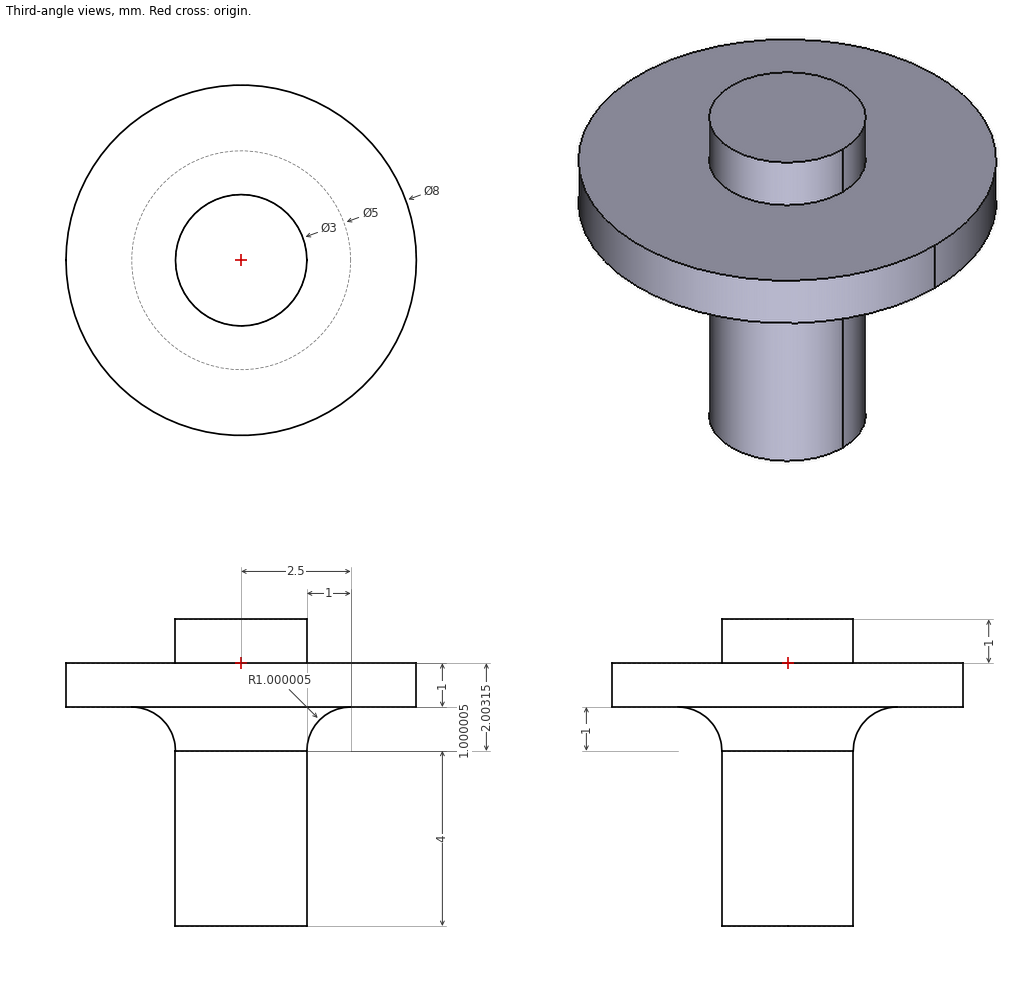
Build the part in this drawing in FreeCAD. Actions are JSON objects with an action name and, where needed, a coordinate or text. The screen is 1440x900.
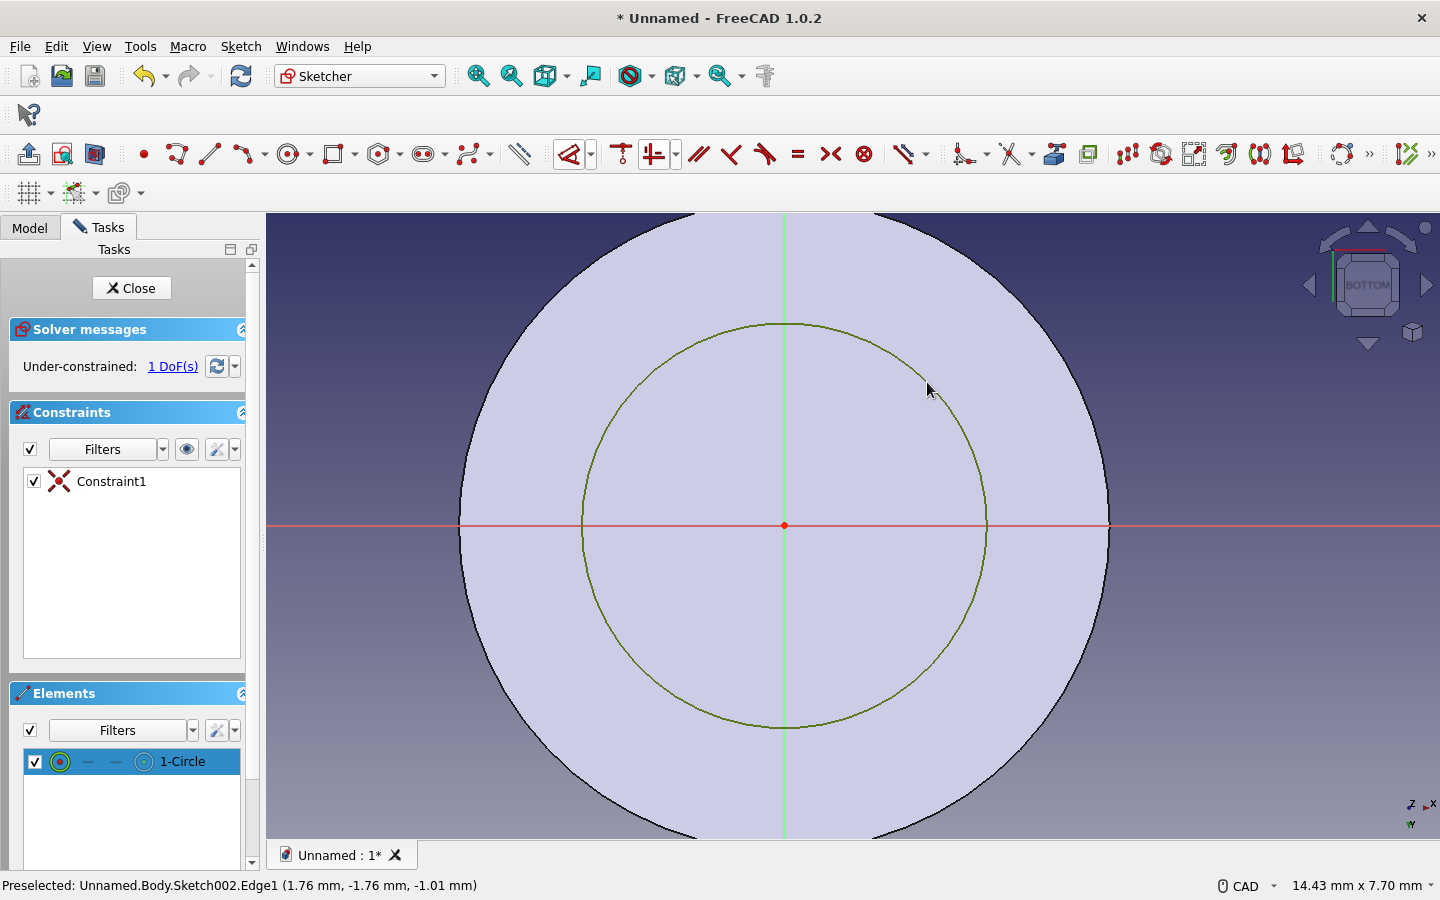
{"action": "key", "text": "k o"}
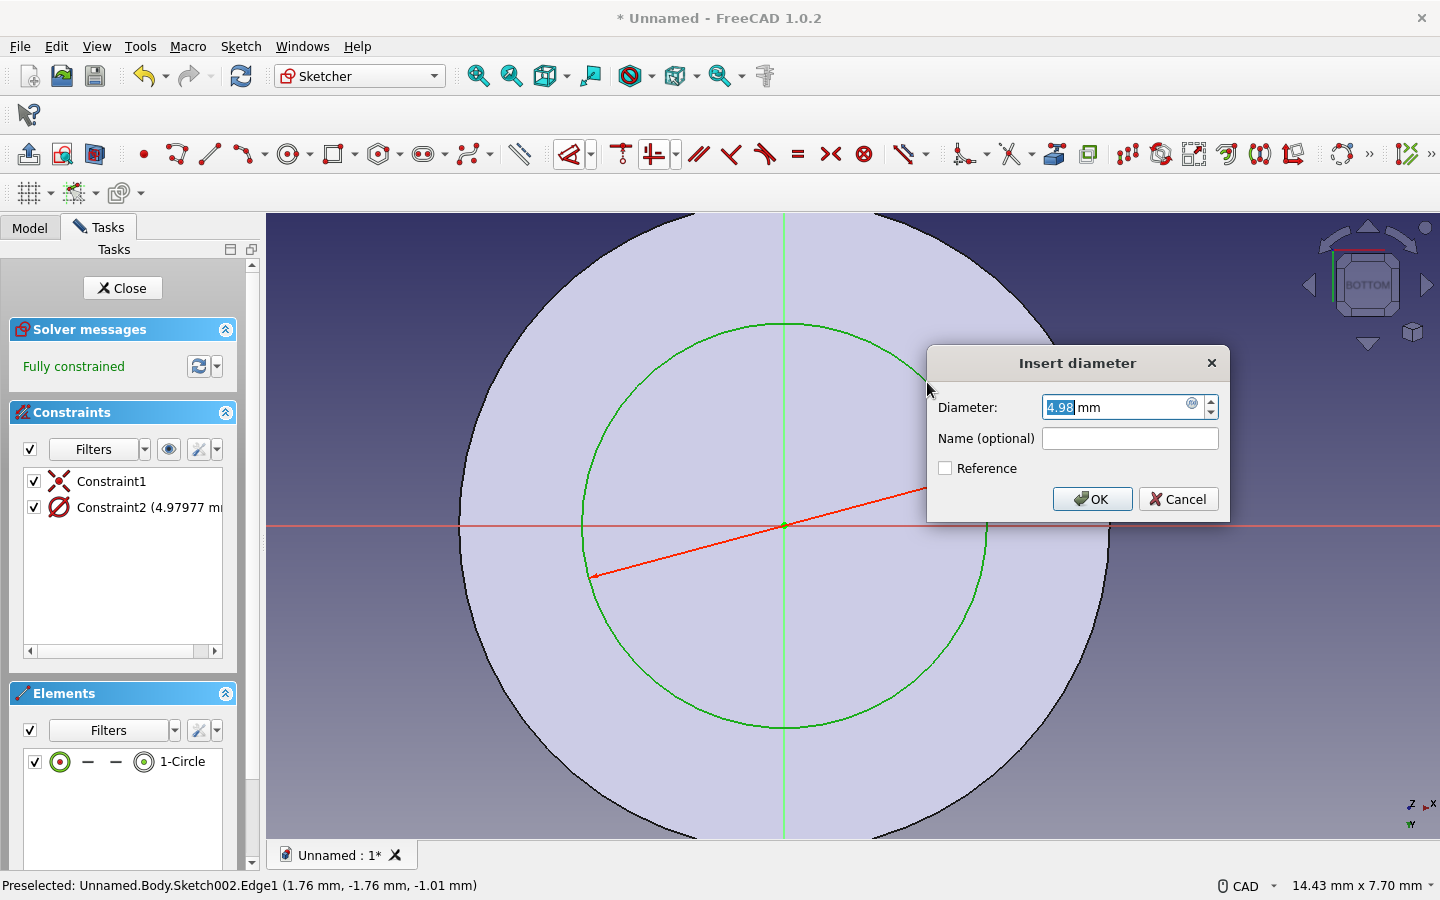
{"action": "type", "text": "5"}
{"action": "key", "text": "Return"}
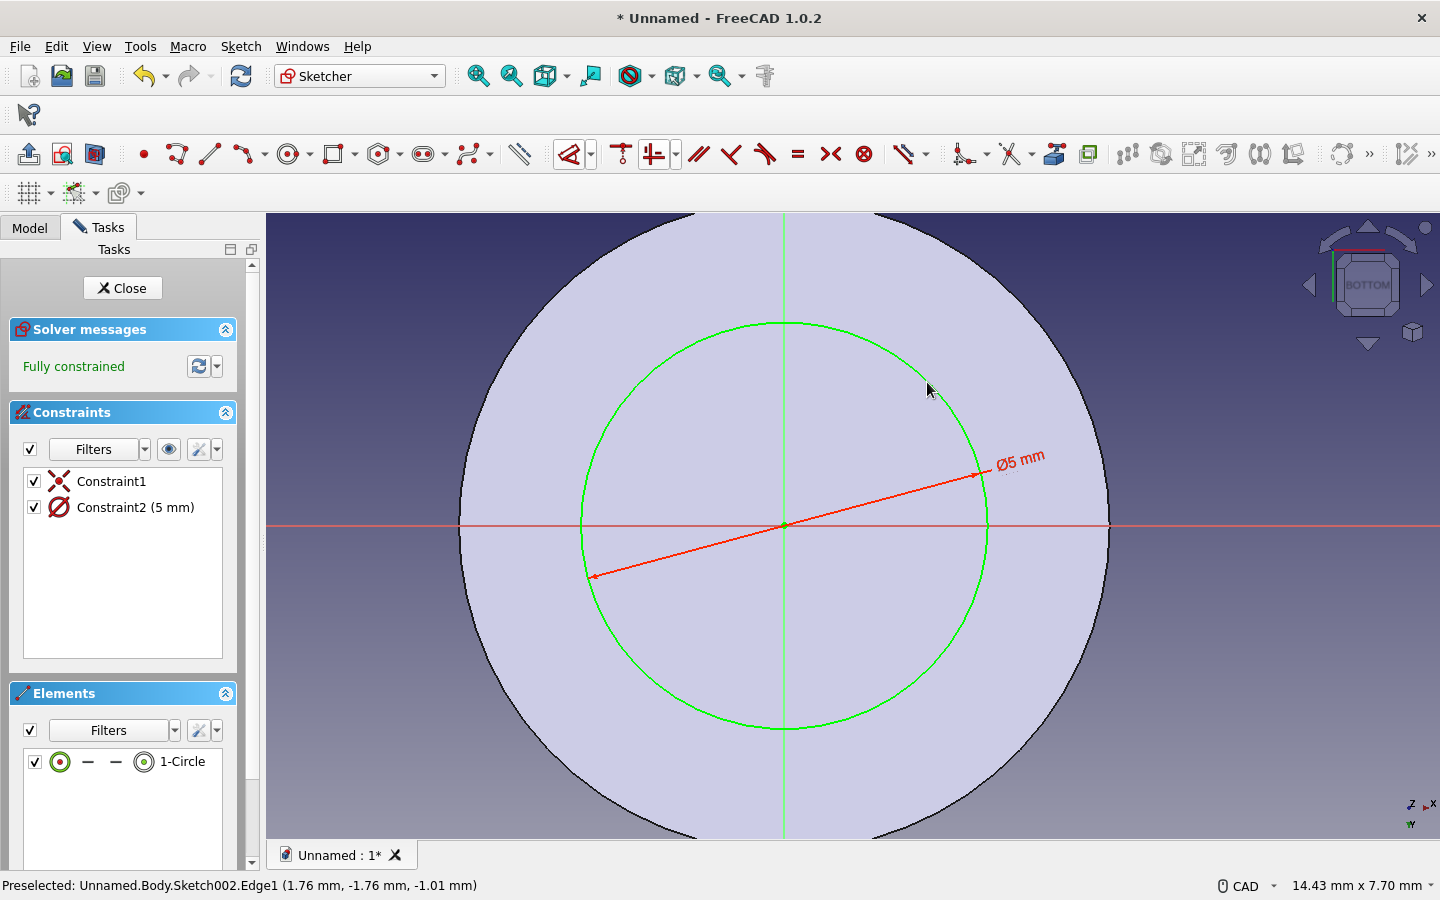
{"action": "left_click", "coordinate": [123, 288]}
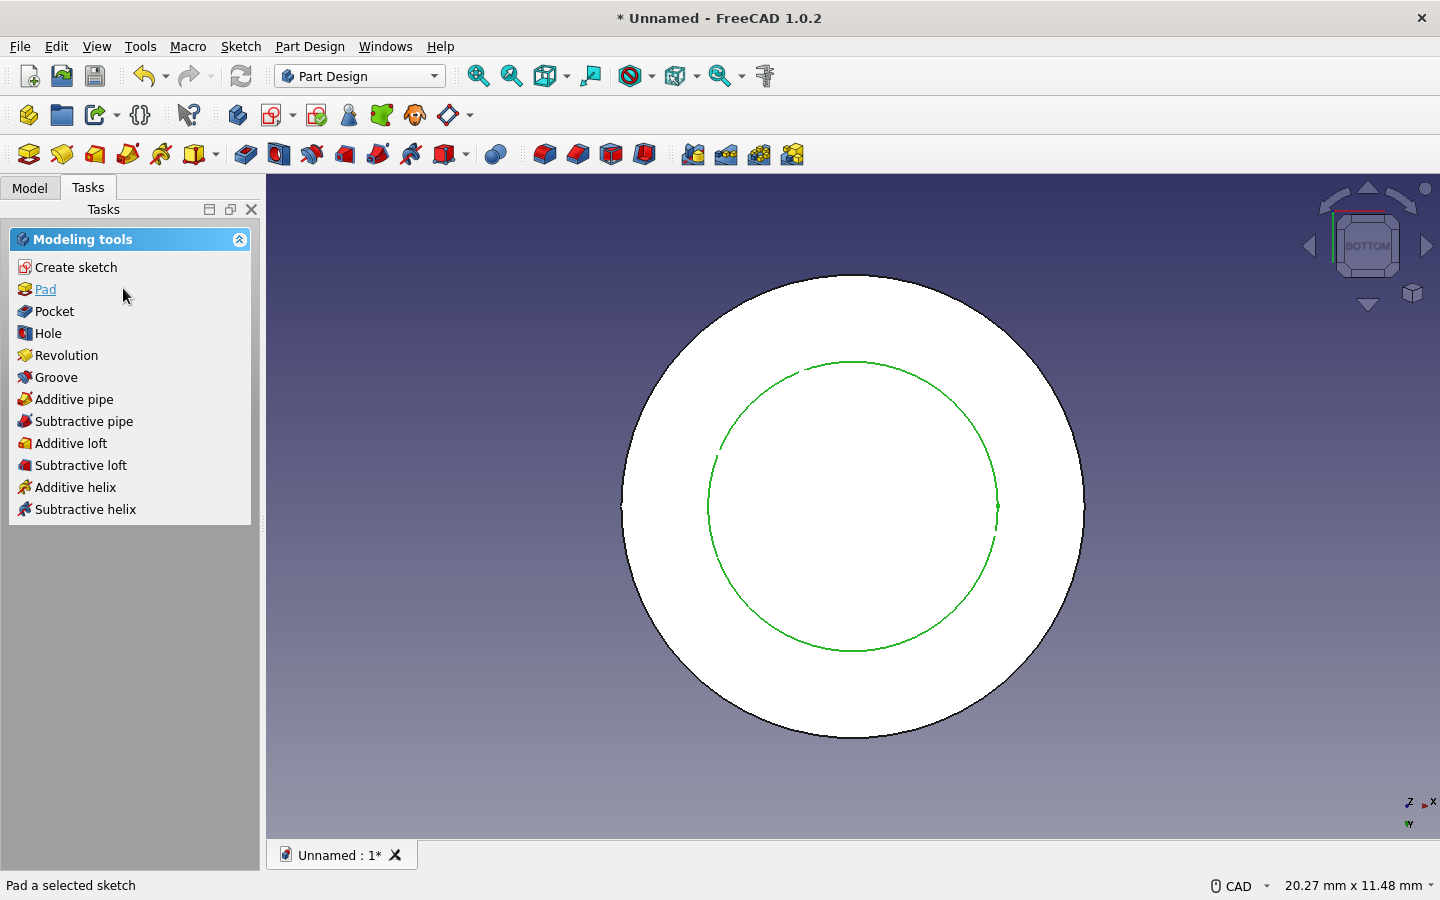
{"action": "left_click", "coordinate": [29, 154]}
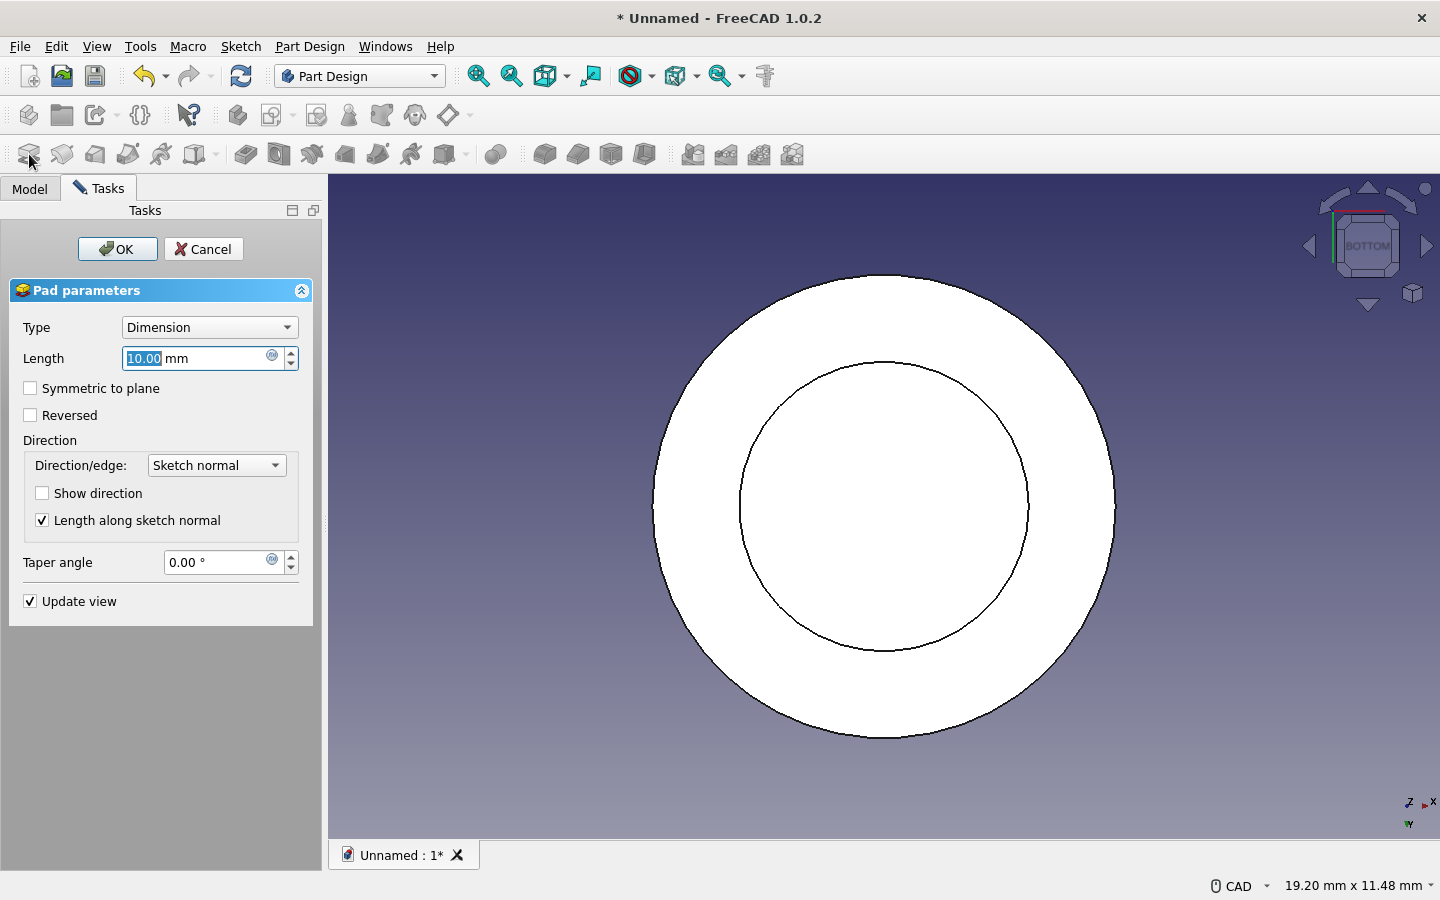
{"action": "type", "text": "1"}
{"action": "key", "text": "Tab"}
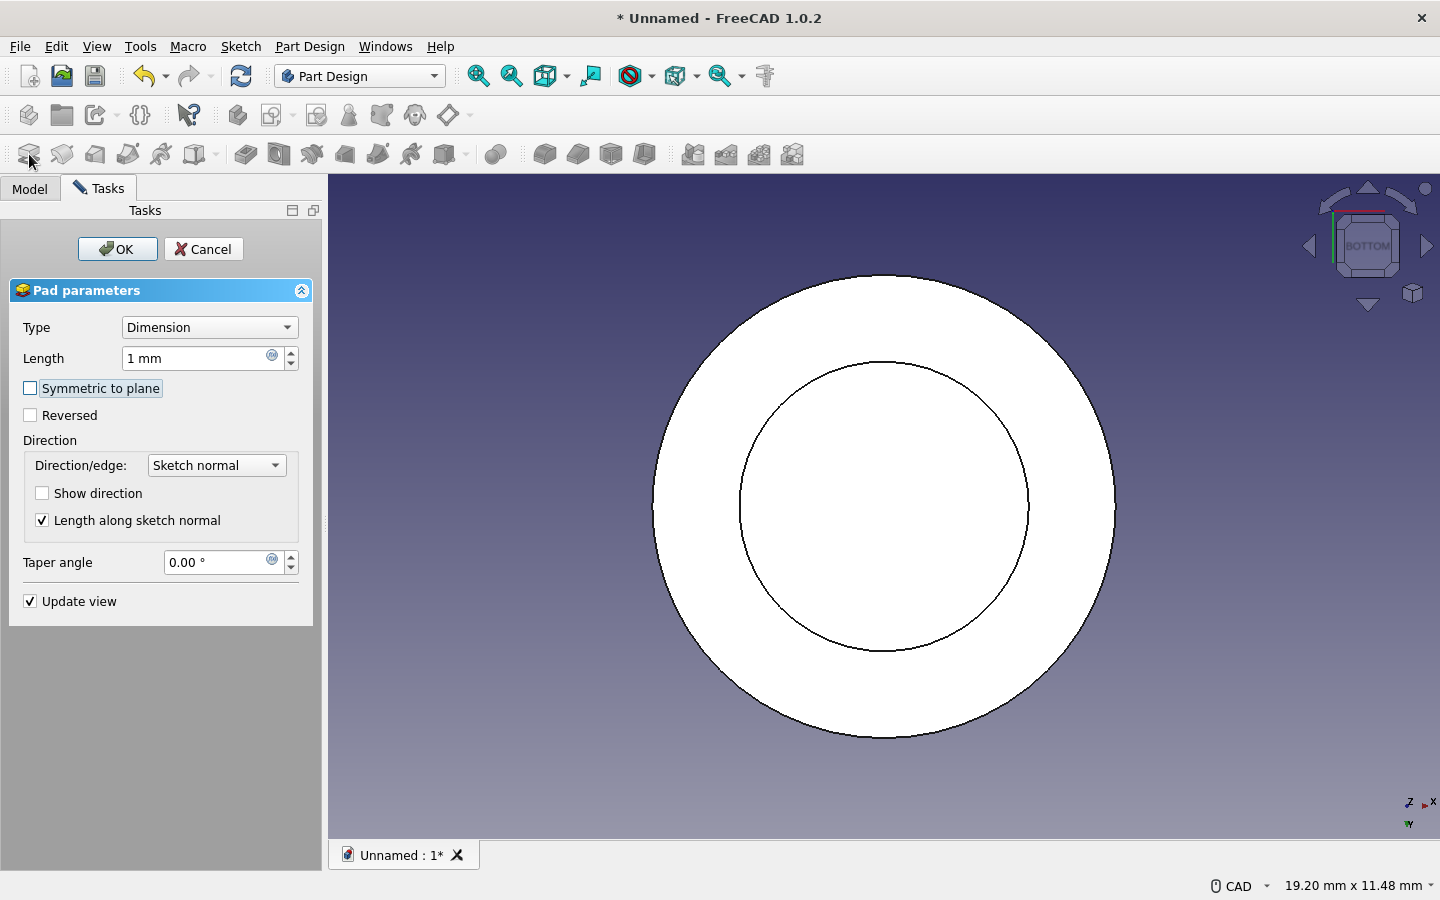
{"action": "left_click", "coordinate": [118, 249]}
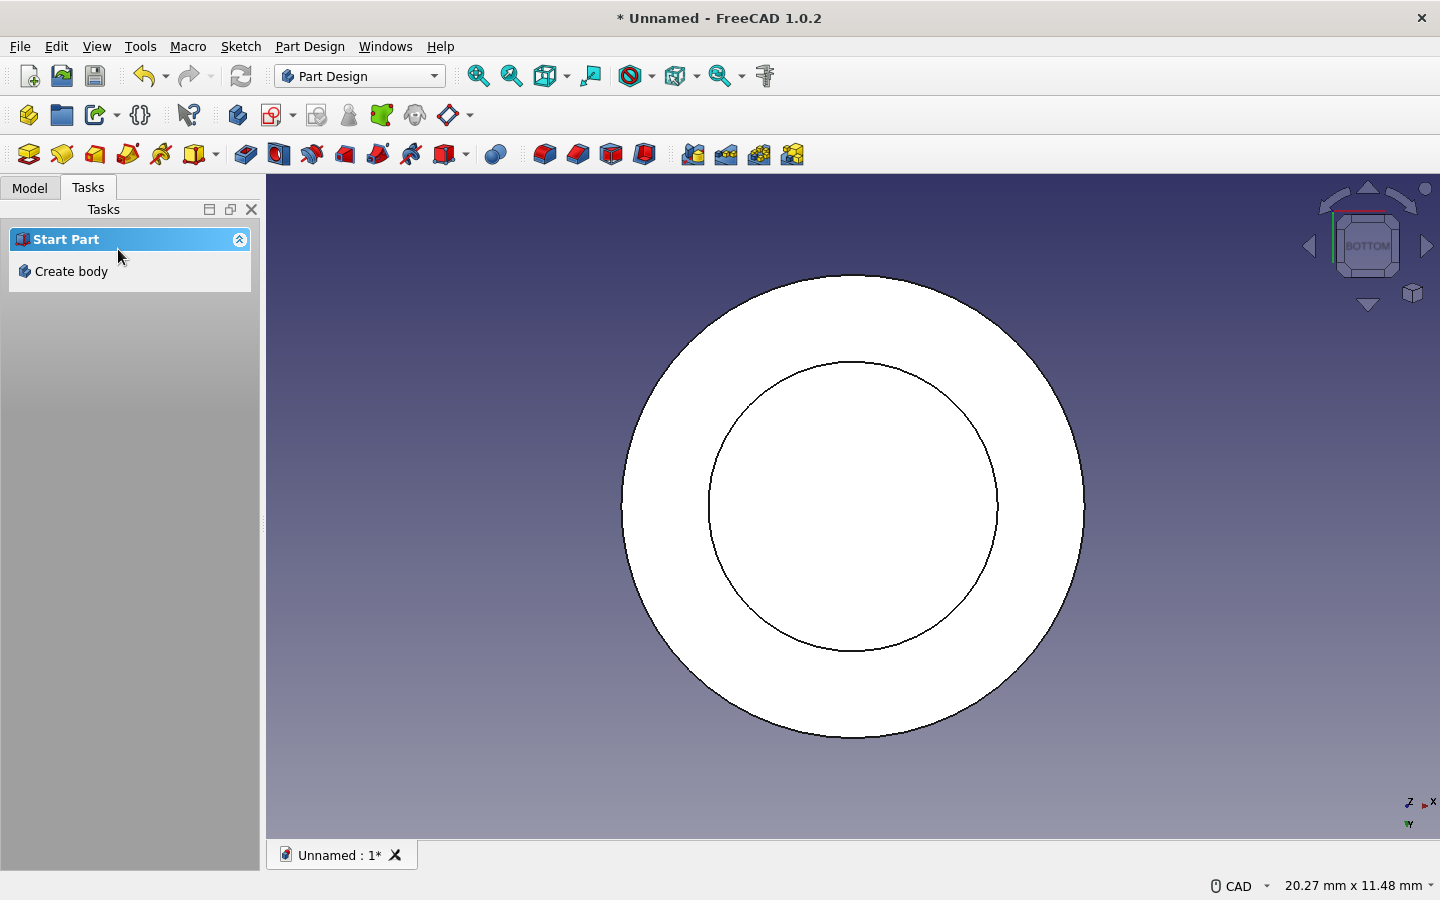
{"action": "left_click", "coordinate": [30, 188]}